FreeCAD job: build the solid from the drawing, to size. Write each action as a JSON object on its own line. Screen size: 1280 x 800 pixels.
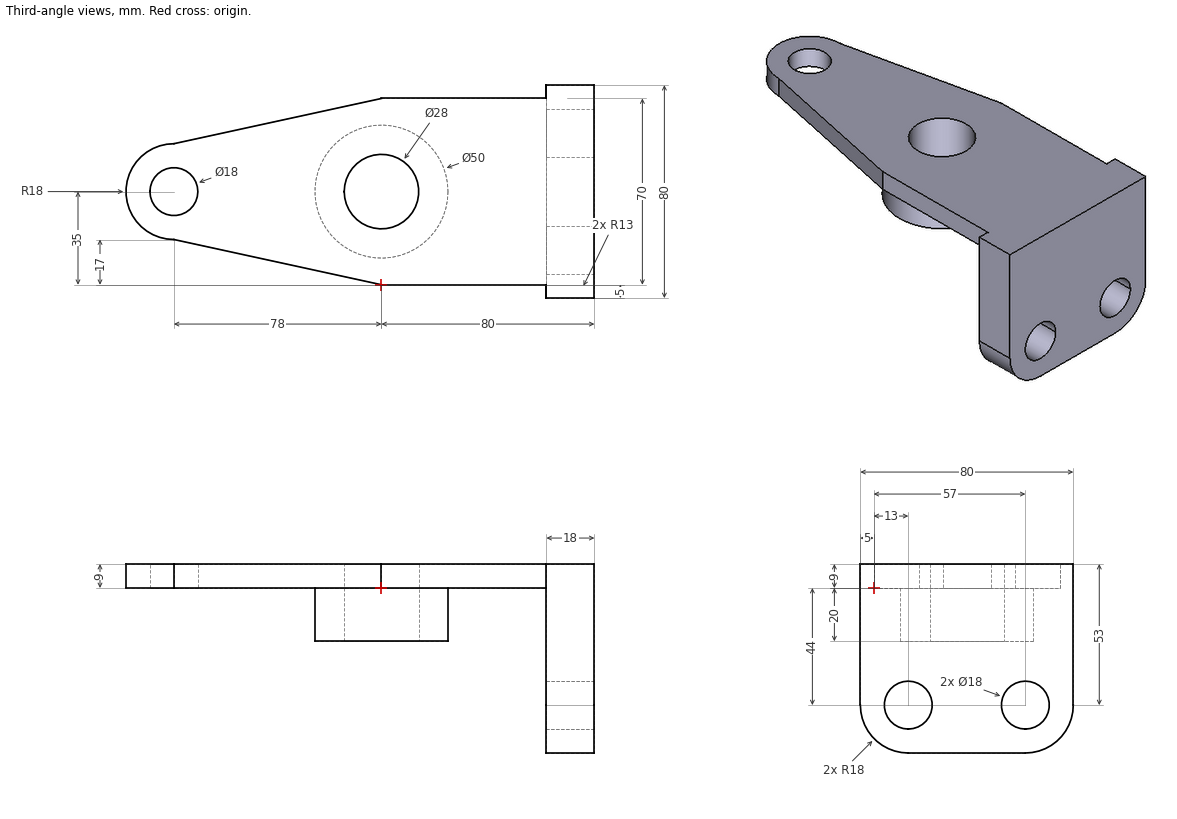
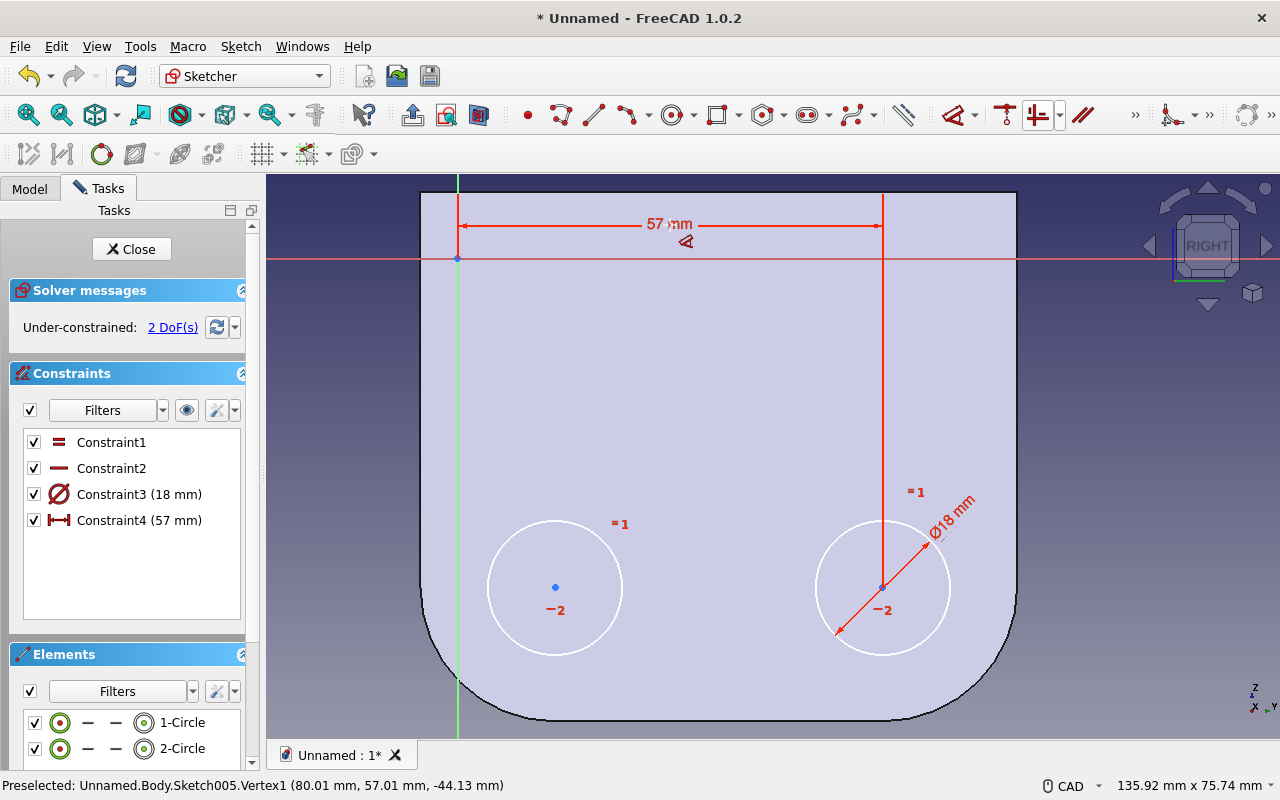
{"action": "left_click", "coordinate": [883, 588]}
{"action": "left_click", "coordinate": [424, 423]}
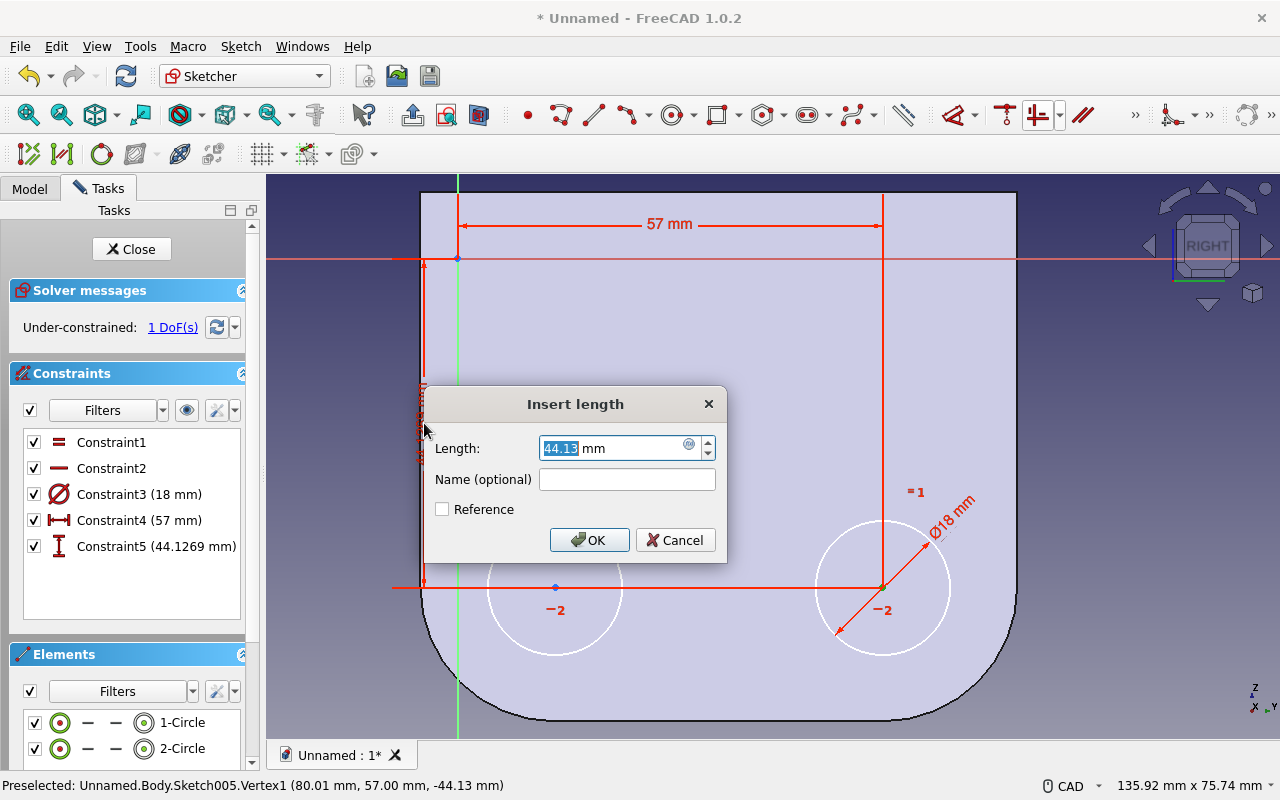
{"action": "type", "text": "44"}
{"action": "key", "text": "Return"}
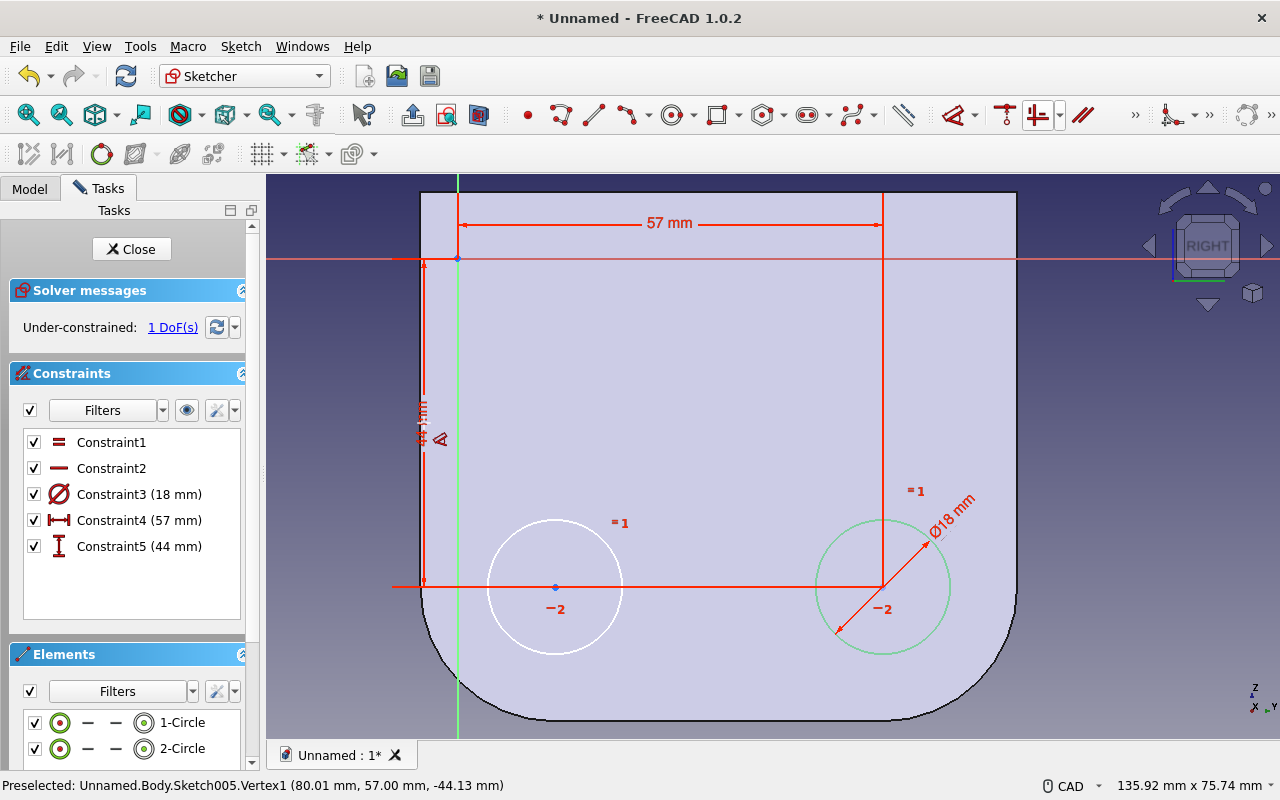
{"action": "left_click", "coordinate": [555, 587]}
{"action": "left_click", "coordinate": [506, 225]}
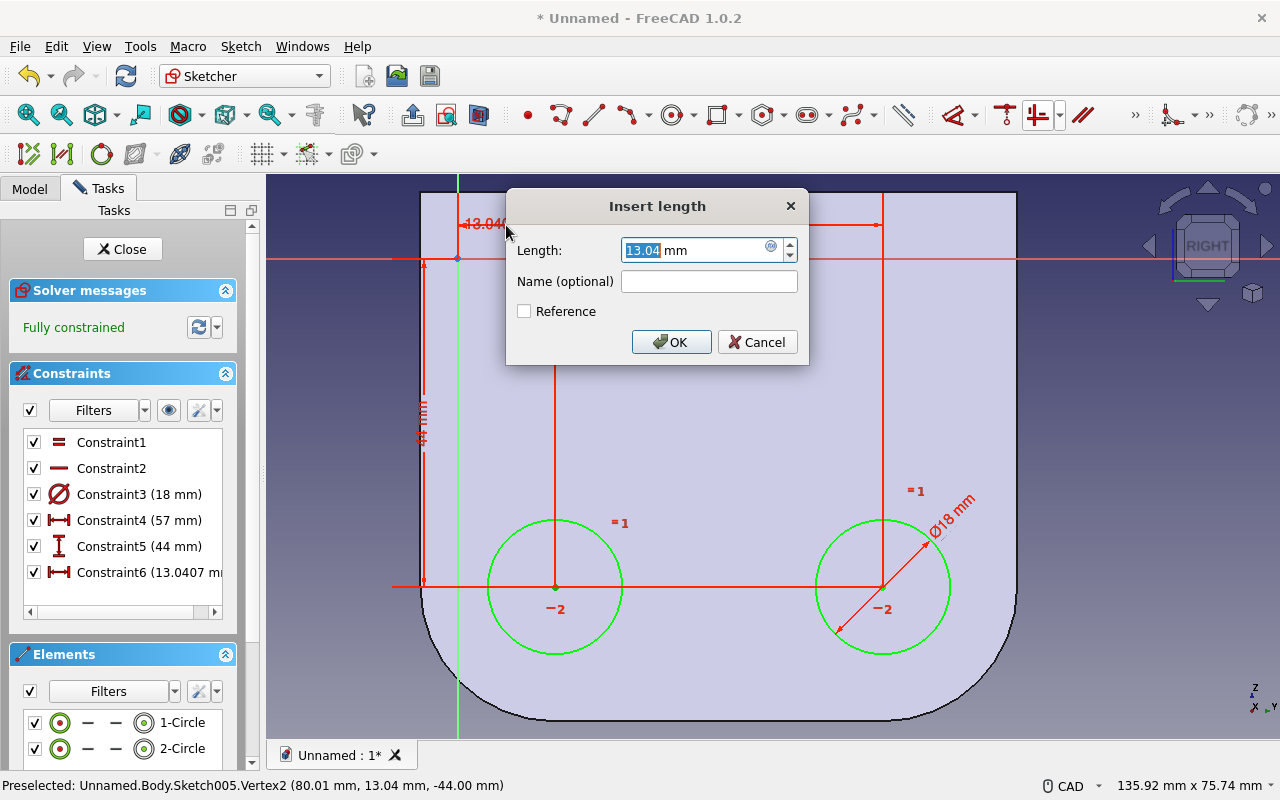
{"action": "type", "text": "13"}
{"action": "key", "text": "Return"}
{"action": "key", "text": "Escape"}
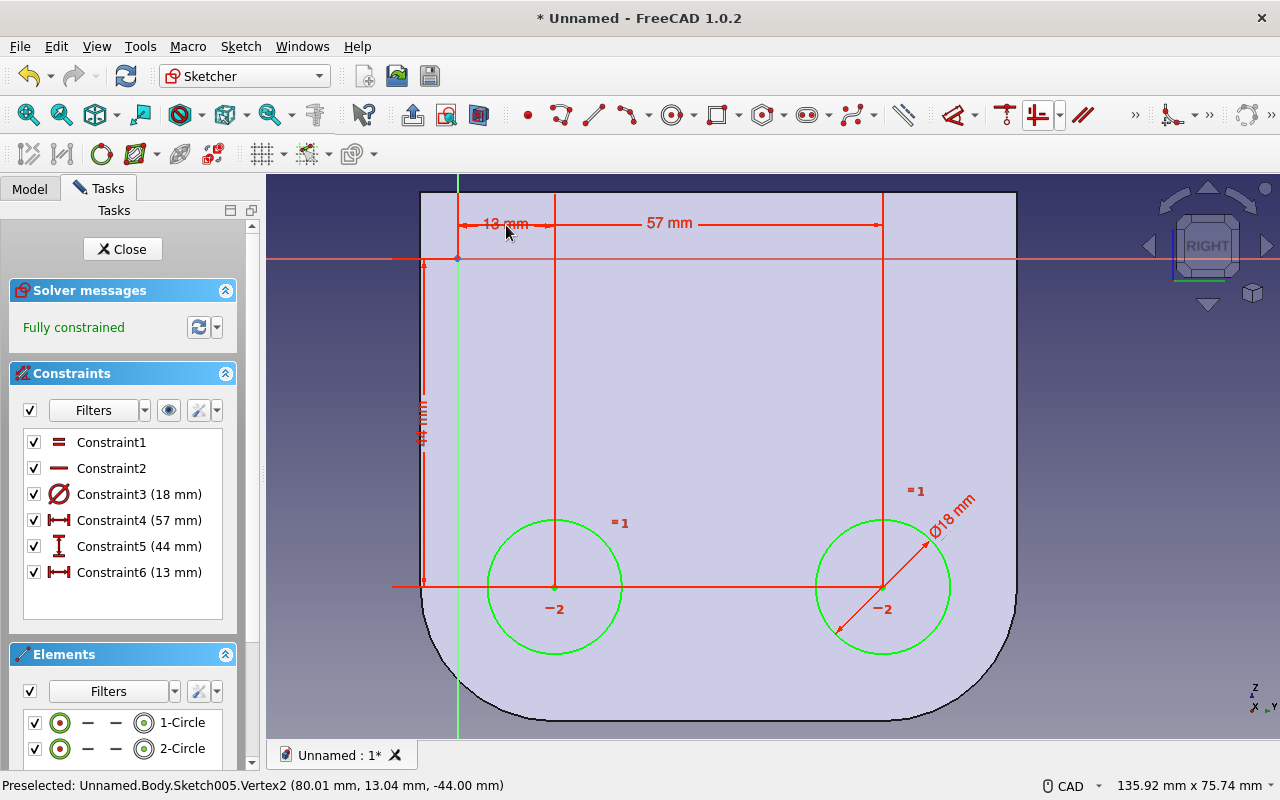
{"action": "left_click", "coordinate": [123, 249]}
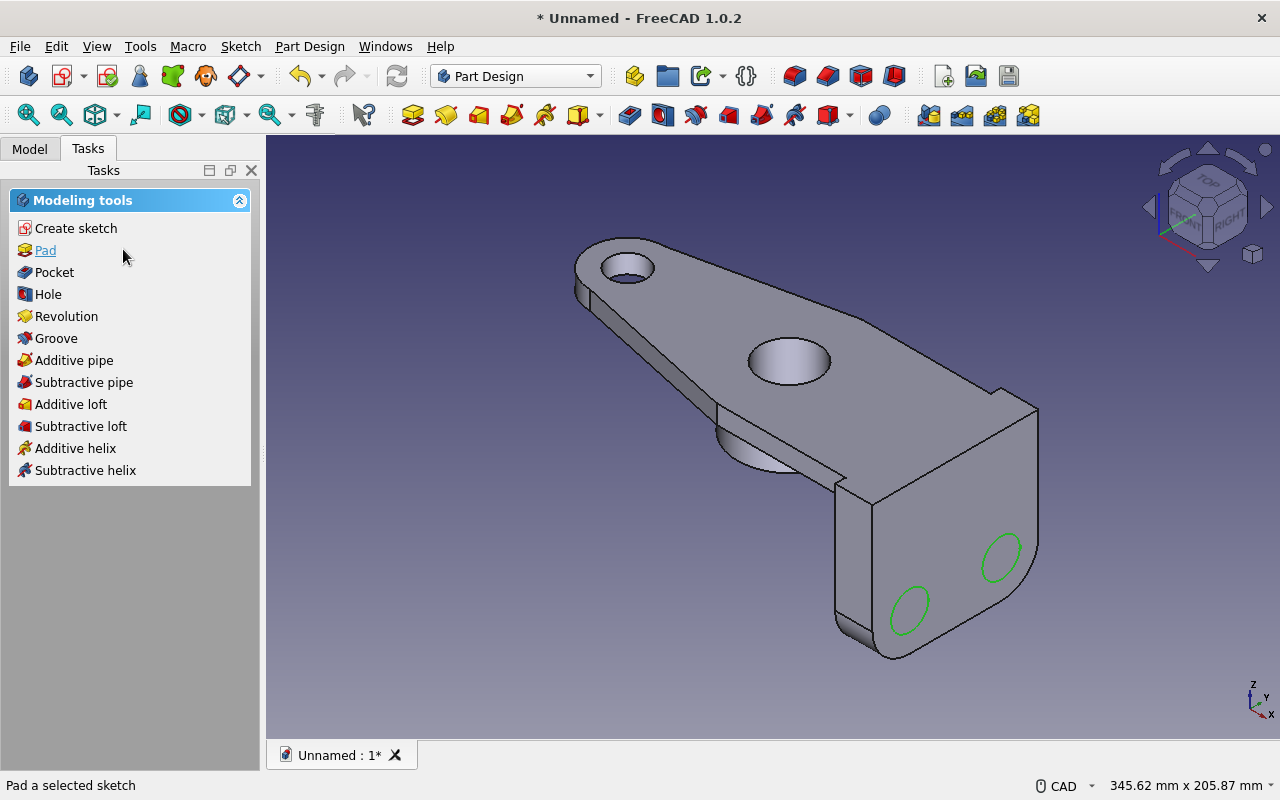
{"action": "left_click", "coordinate": [630, 116]}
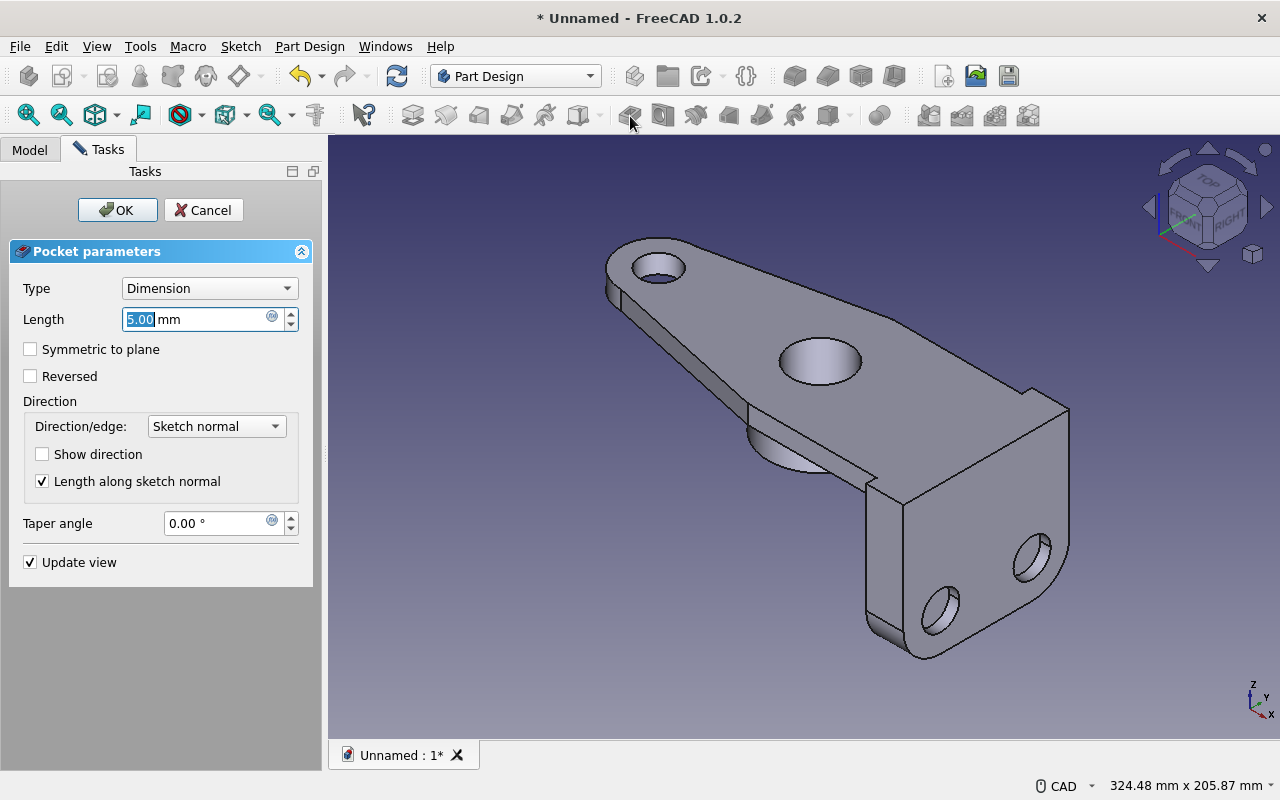
{"action": "type", "text": "18"}
{"action": "key", "text": "Tab"}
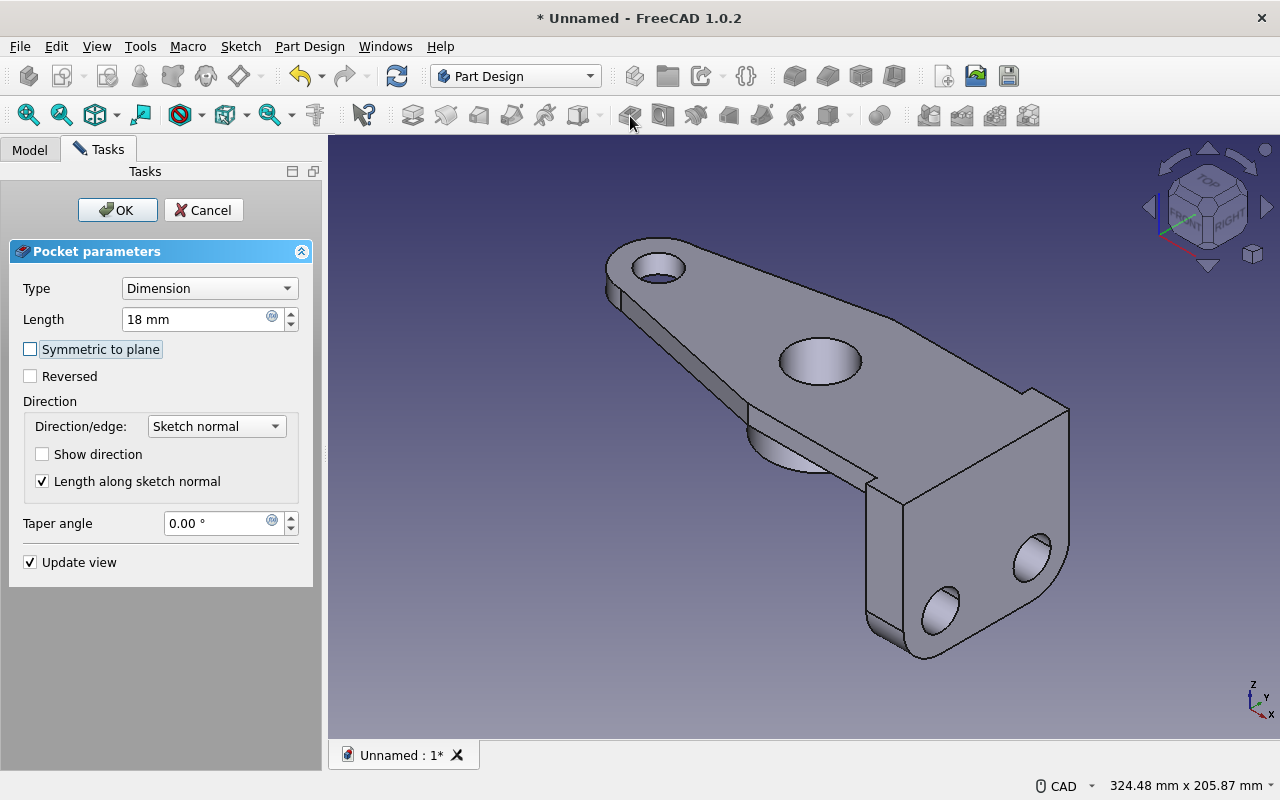
{"action": "left_click", "coordinate": [118, 210]}